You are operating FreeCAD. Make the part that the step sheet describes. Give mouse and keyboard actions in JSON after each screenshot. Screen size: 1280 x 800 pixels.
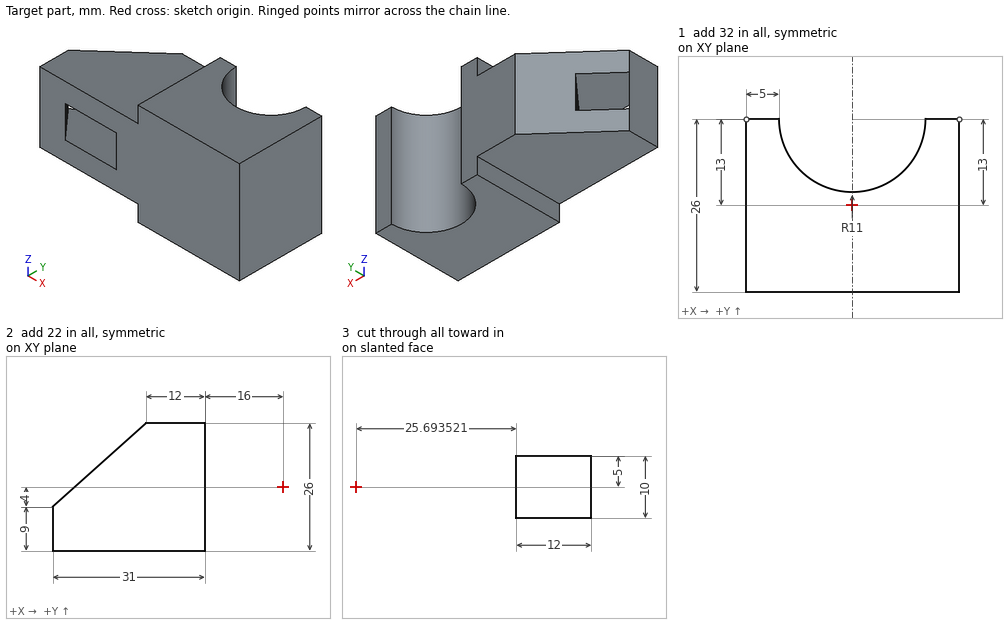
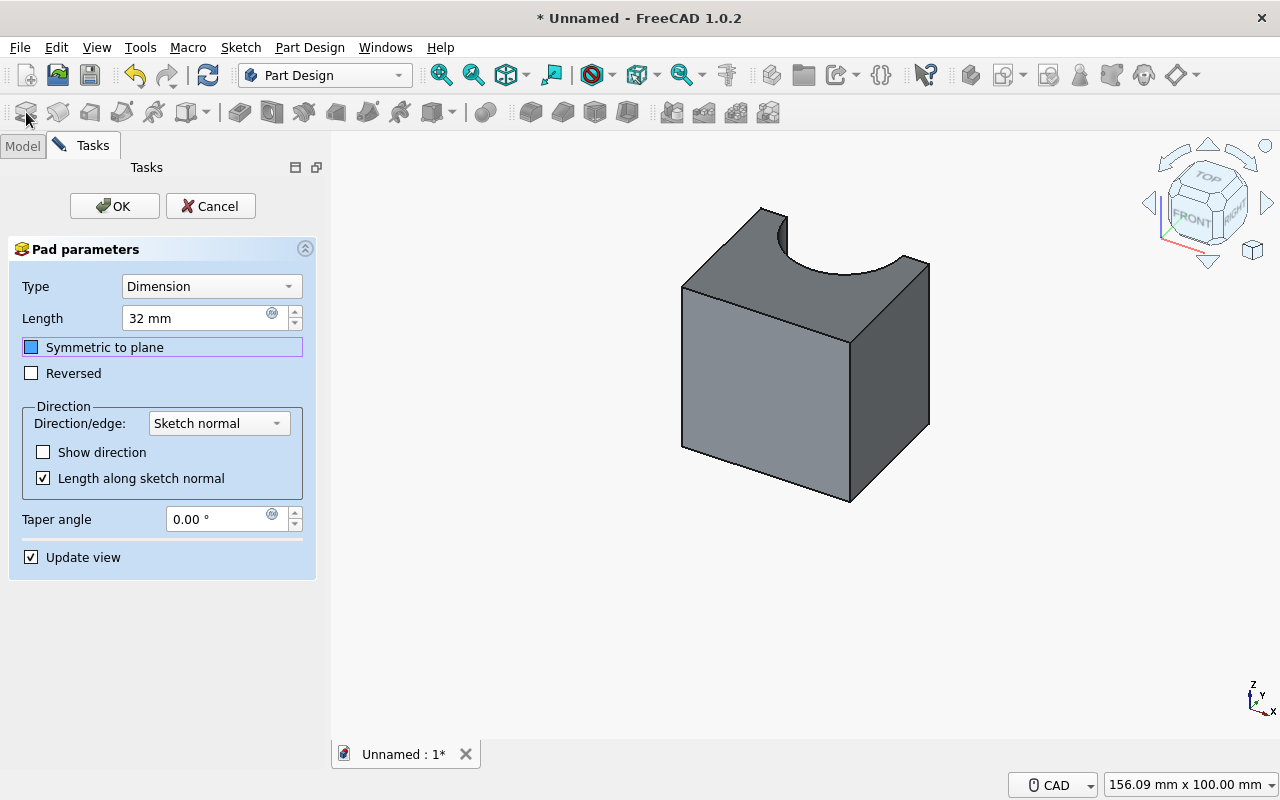
{"action": "left_click", "coordinate": [30, 347]}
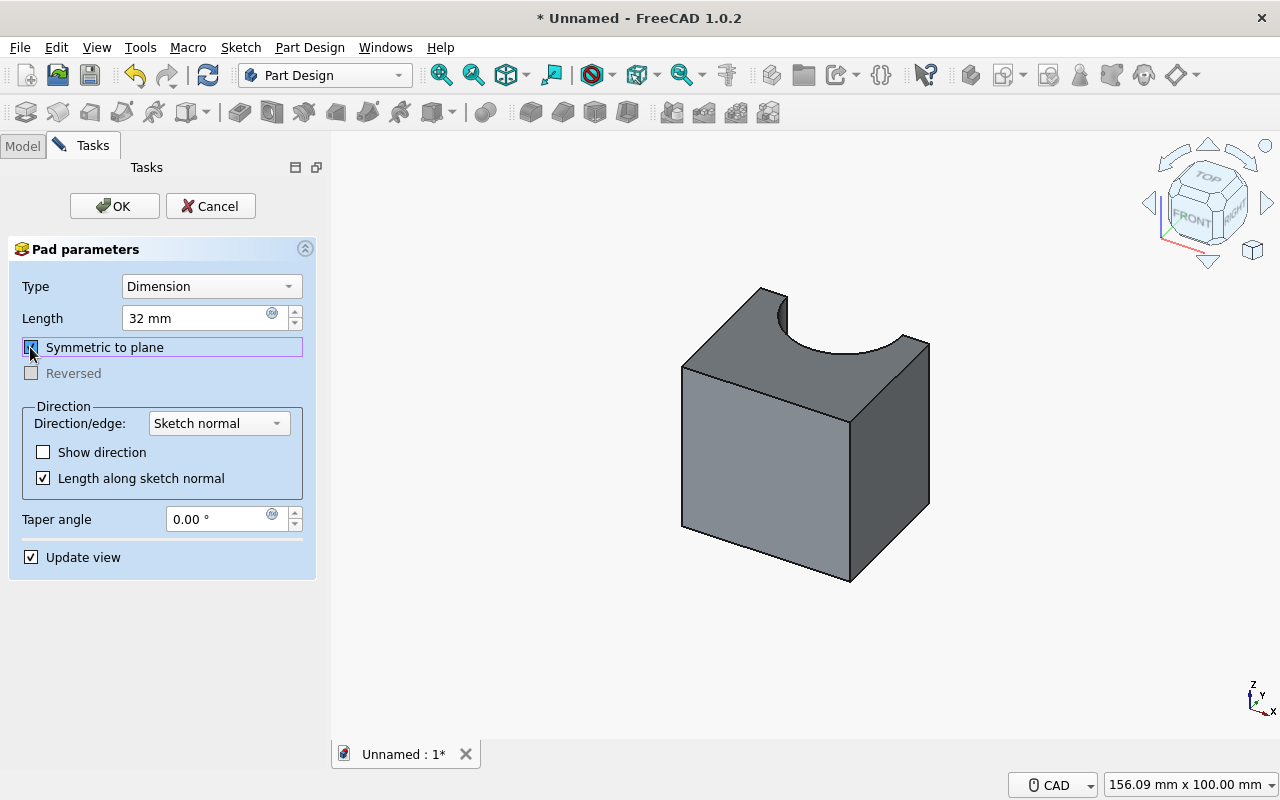
{"action": "left_click", "coordinate": [115, 206]}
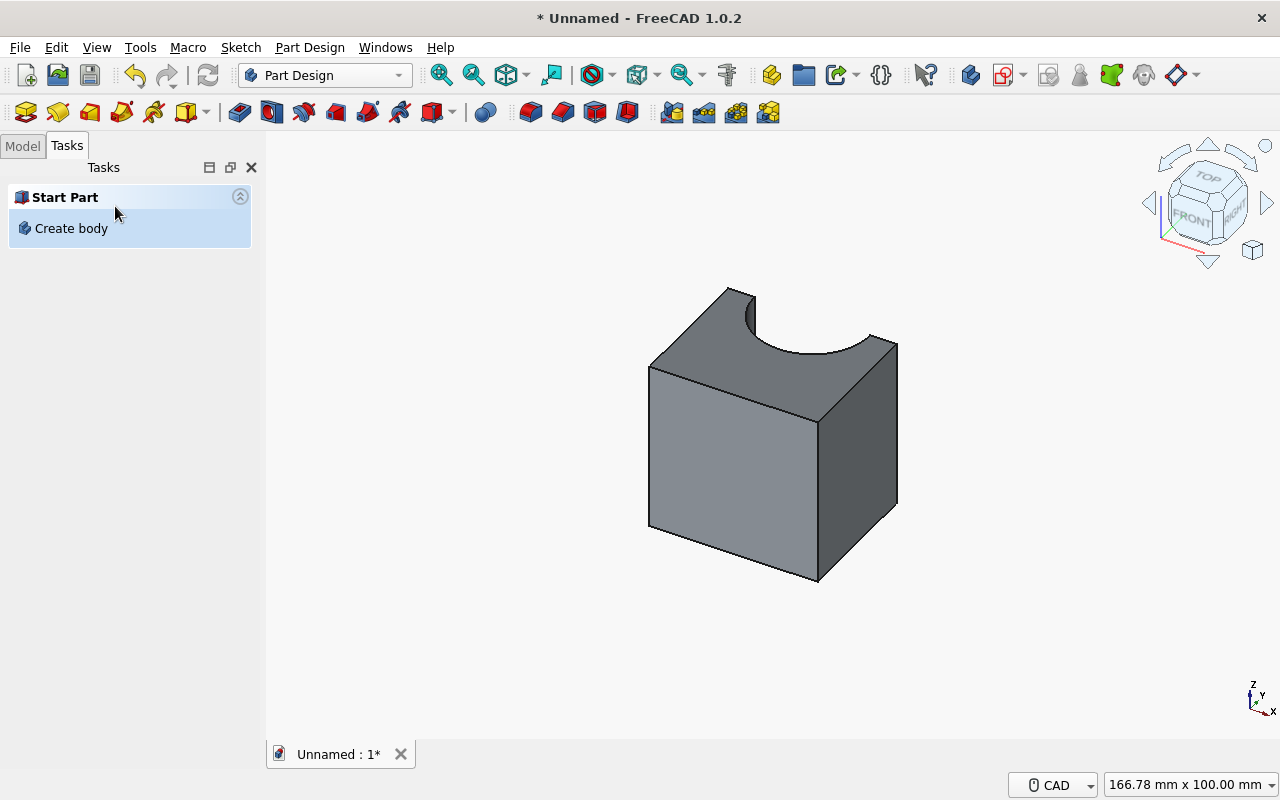
{"action": "left_click", "coordinate": [1004, 76]}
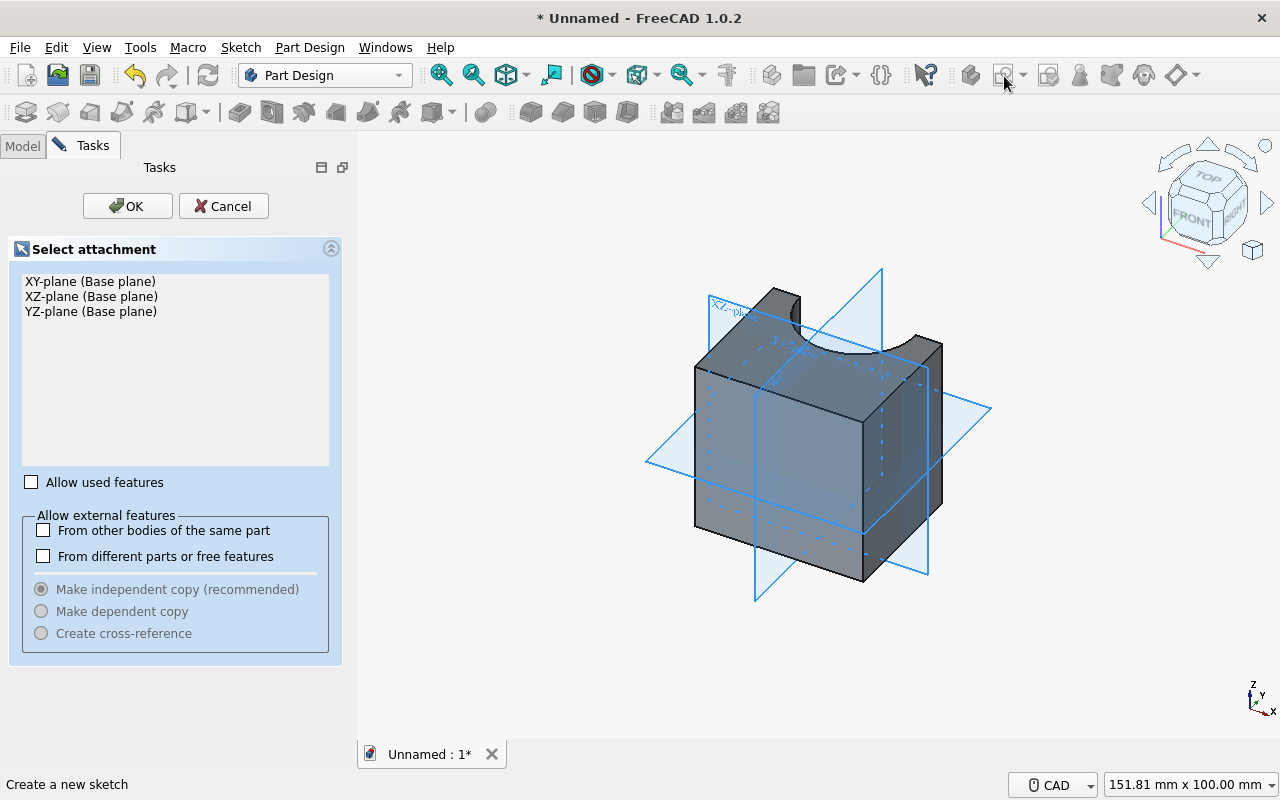
{"action": "left_click", "coordinate": [82, 282]}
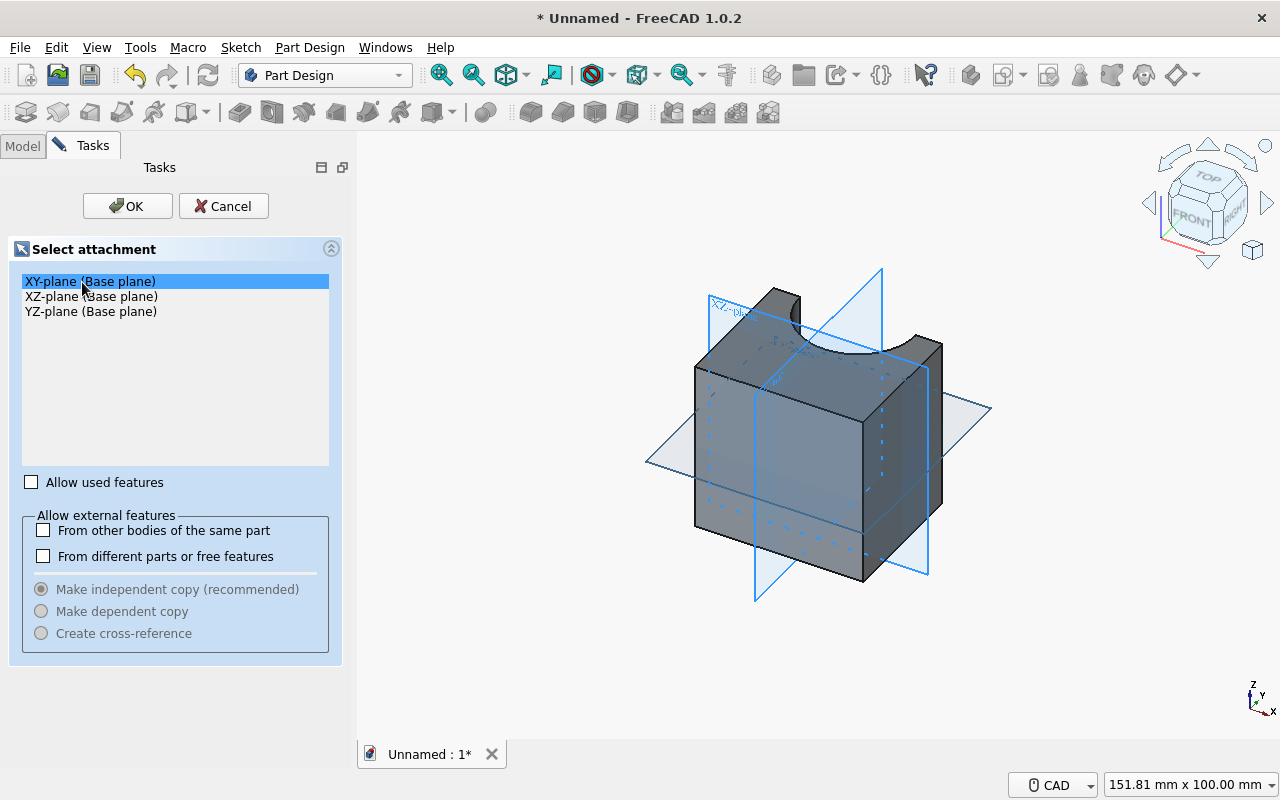
{"action": "left_click", "coordinate": [128, 206]}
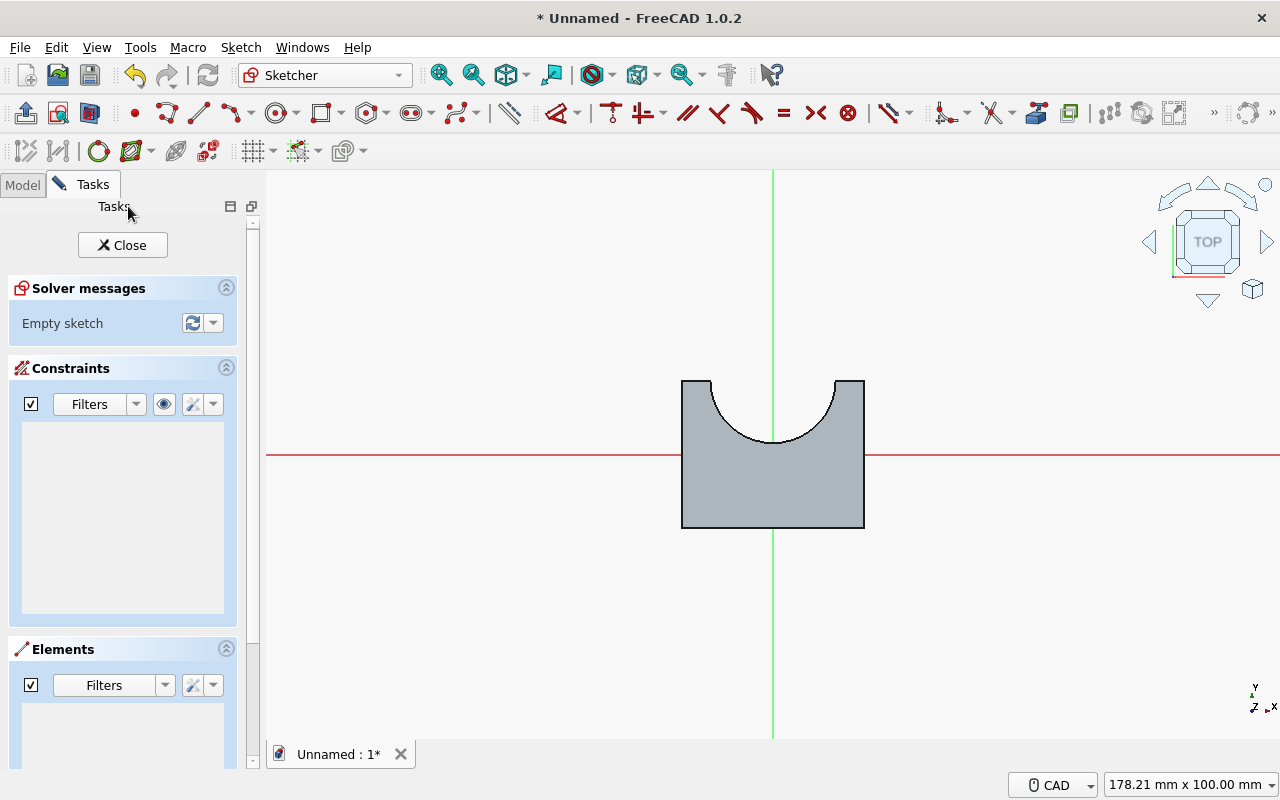
{"action": "key", "text": "q s"}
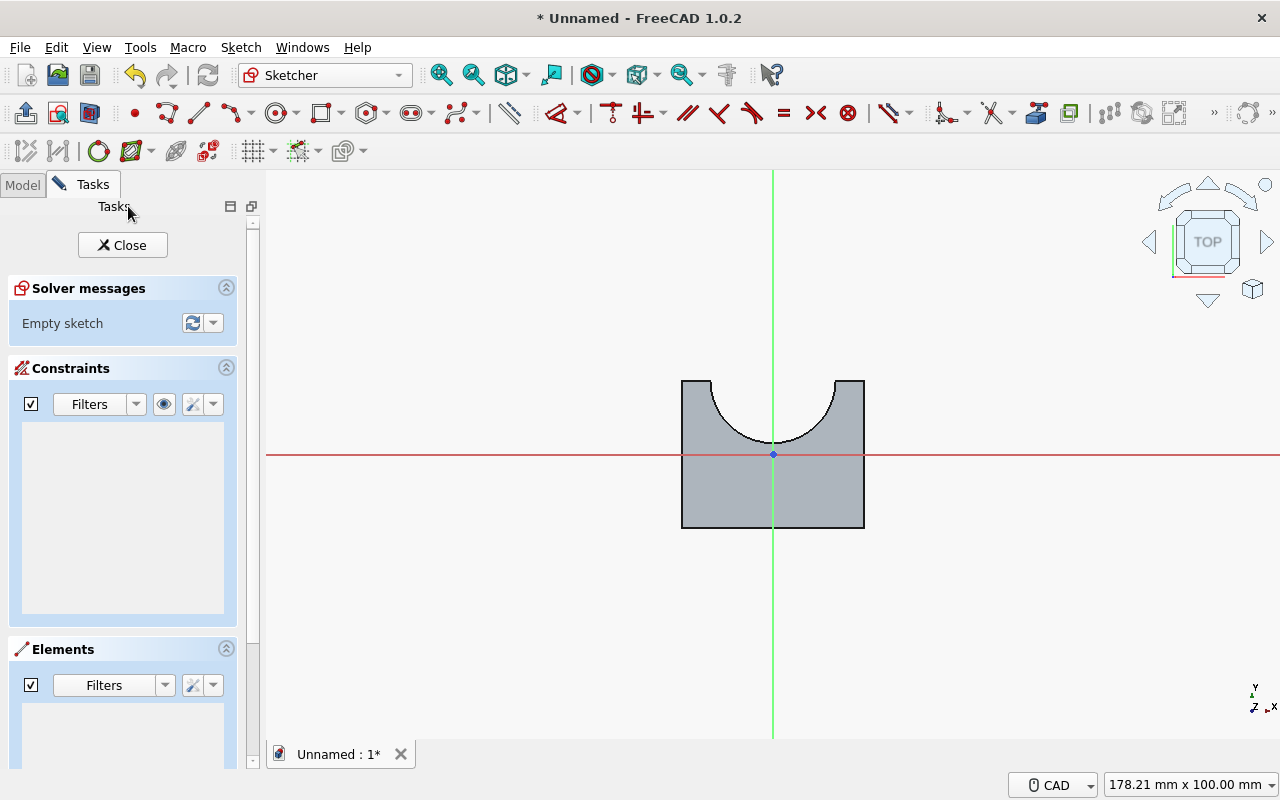
{"action": "scroll", "coordinate": [586, 455], "scroll_direction": "up", "scroll_amount": 4}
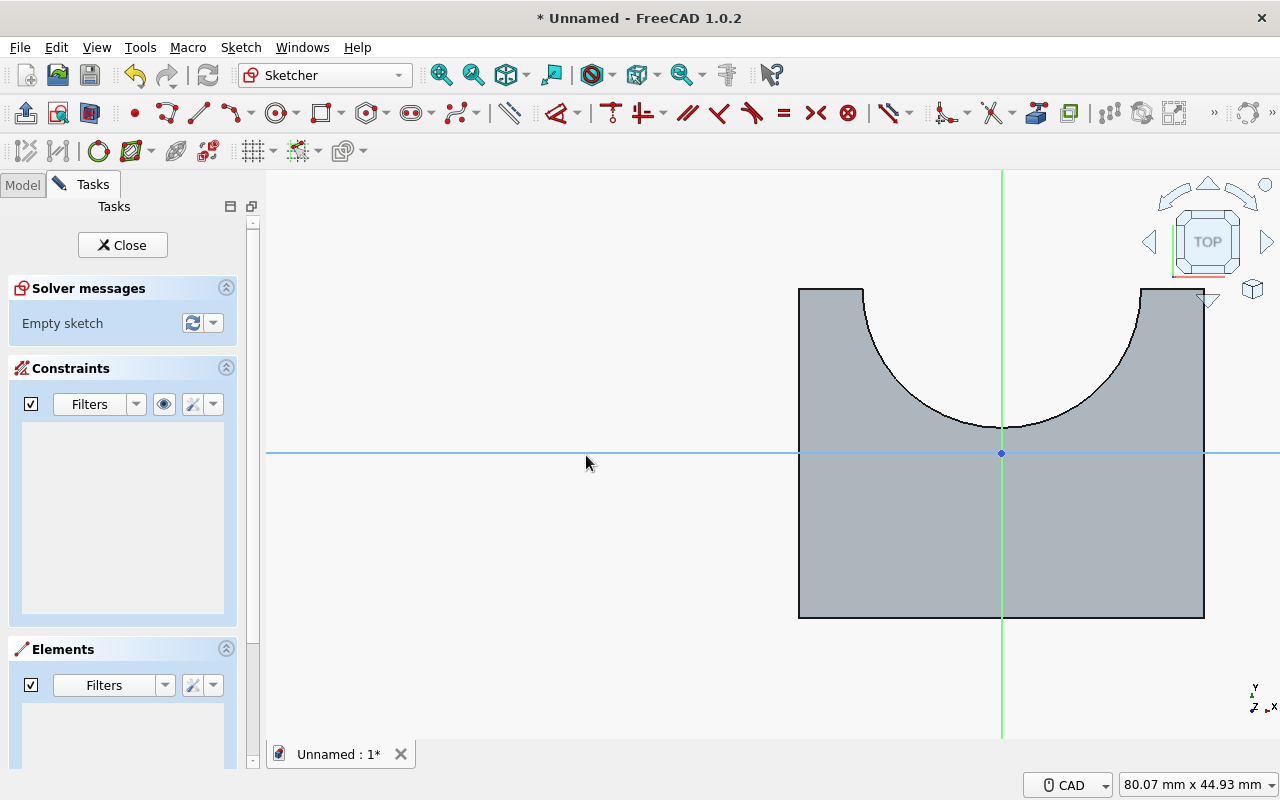
{"action": "key", "text": "g m"}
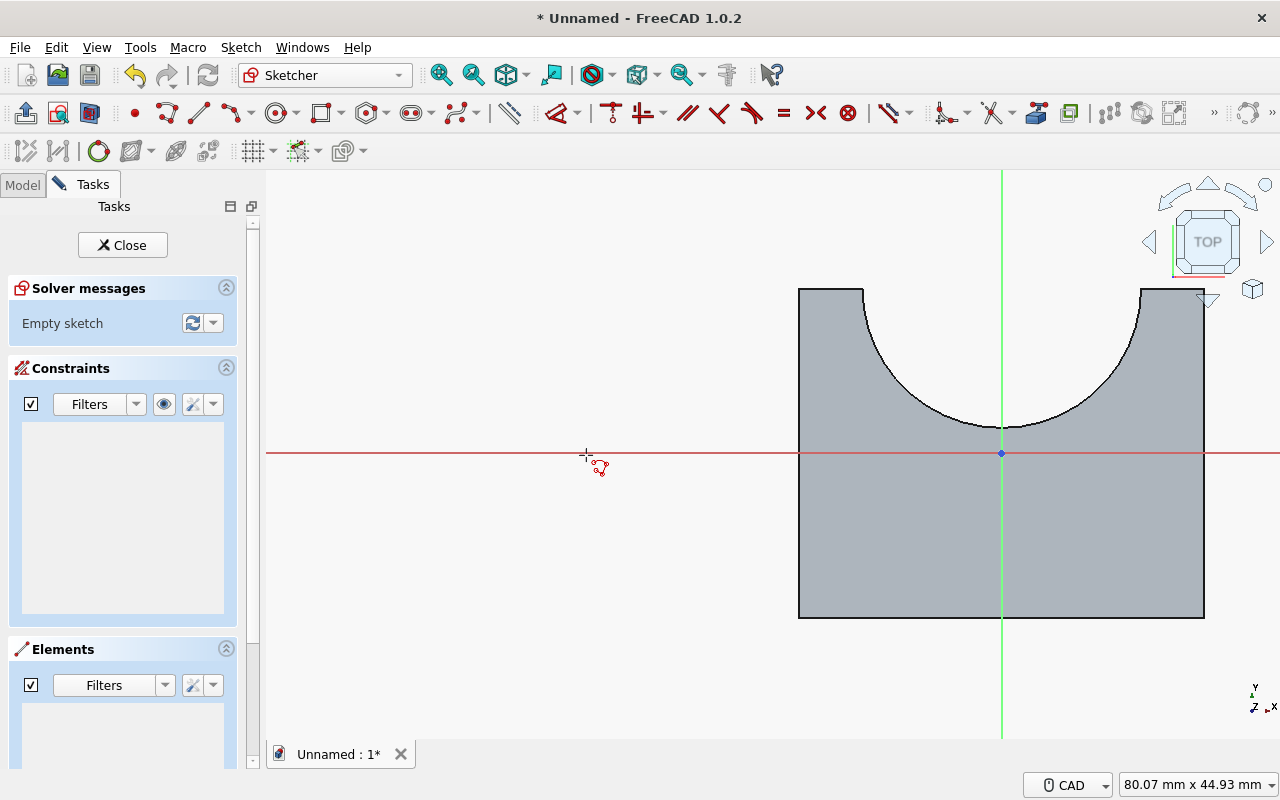
{"action": "left_click", "coordinate": [799, 289]}
{"action": "left_click", "coordinate": [647, 289]}
{"action": "left_click", "coordinate": [407, 504]}
{"action": "left_click", "coordinate": [407, 618]}
{"action": "left_click", "coordinate": [799, 618]}
{"action": "left_click", "coordinate": [799, 290]}
{"action": "key", "text": "Escape"}
{"action": "key", "text": "Escape"}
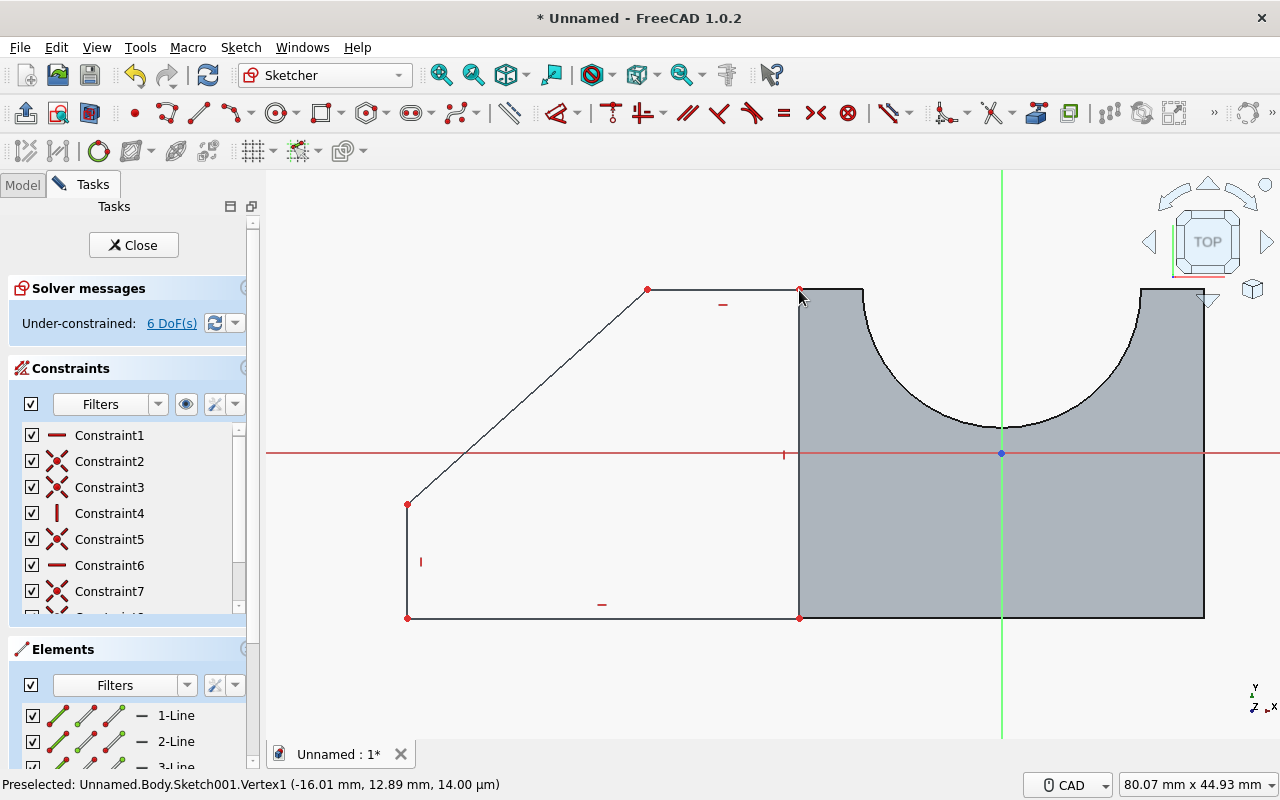
{"action": "key", "text": "d"}